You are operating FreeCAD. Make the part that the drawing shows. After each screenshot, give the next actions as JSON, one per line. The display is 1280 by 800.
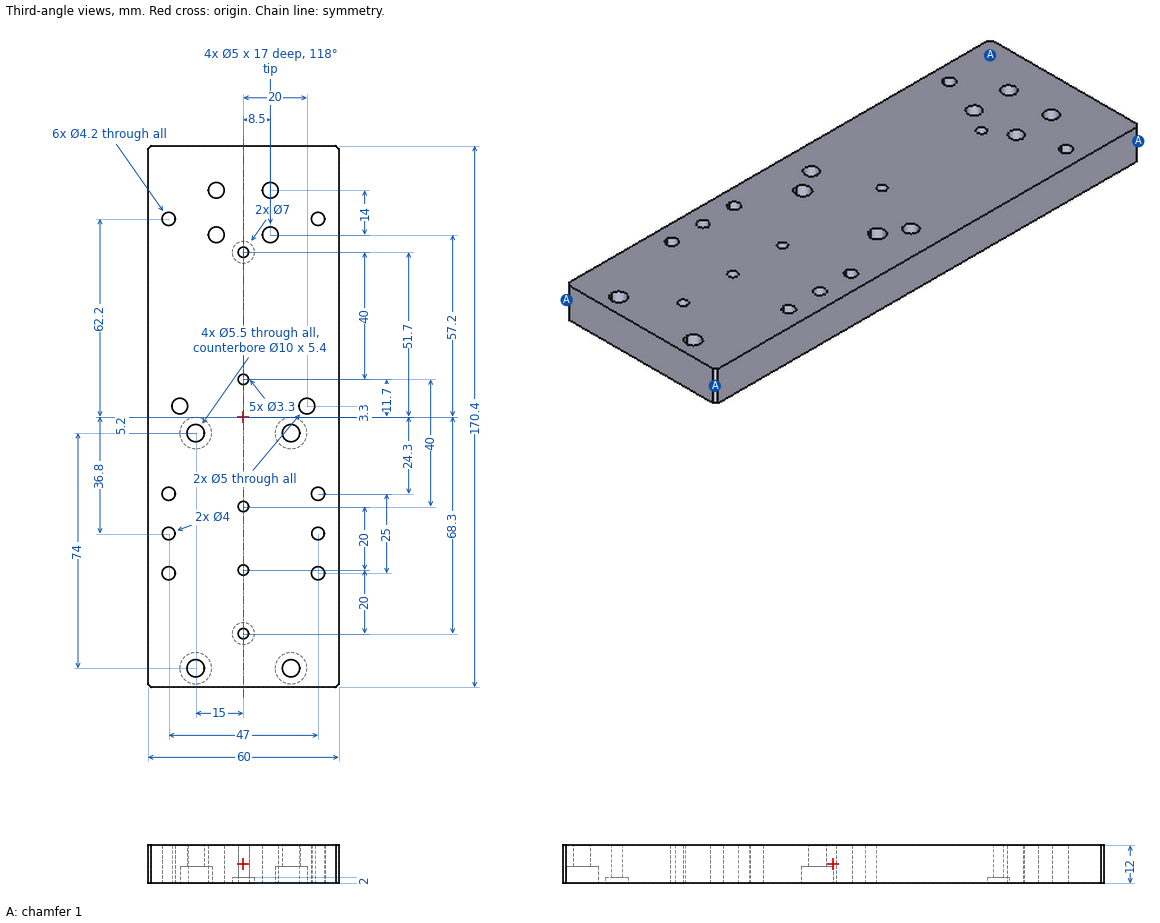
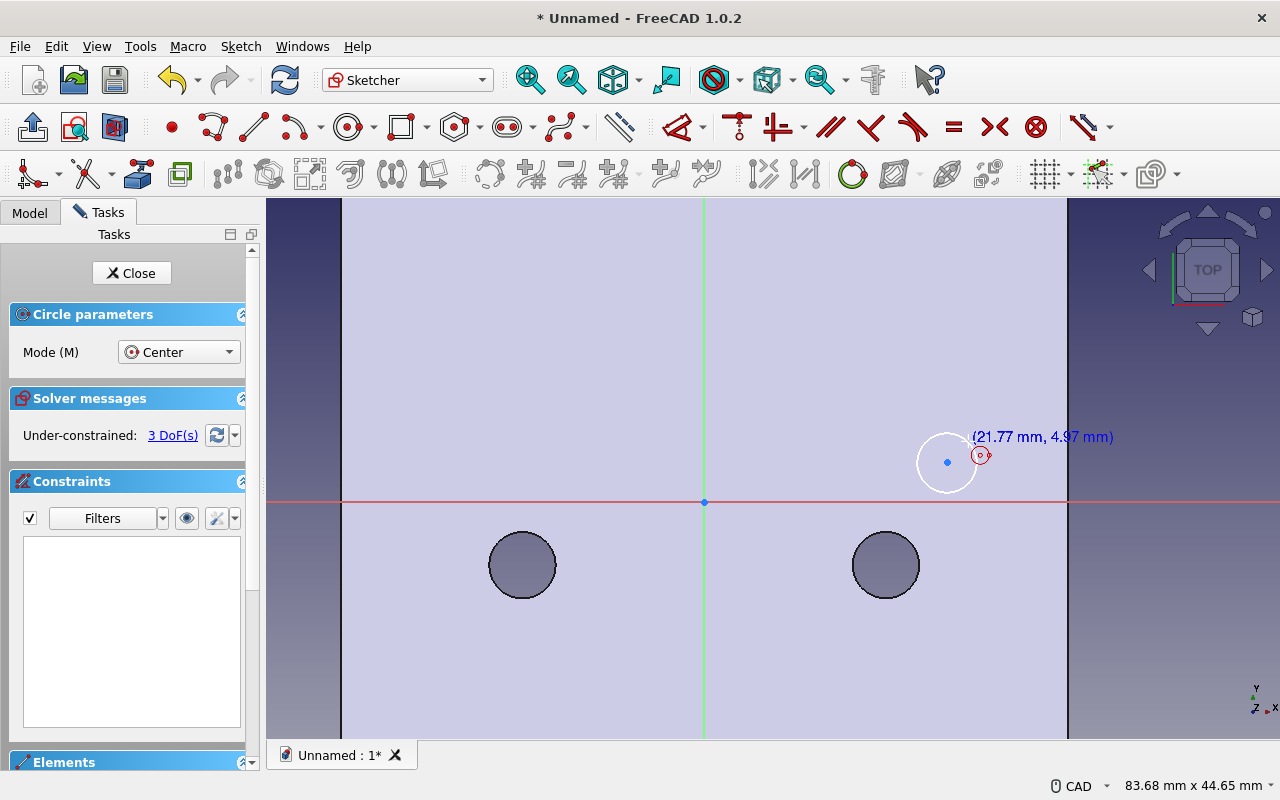
{"action": "left_click", "coordinate": [462, 462]}
{"action": "left_click", "coordinate": [483, 441]}
{"action": "key", "text": "Escape"}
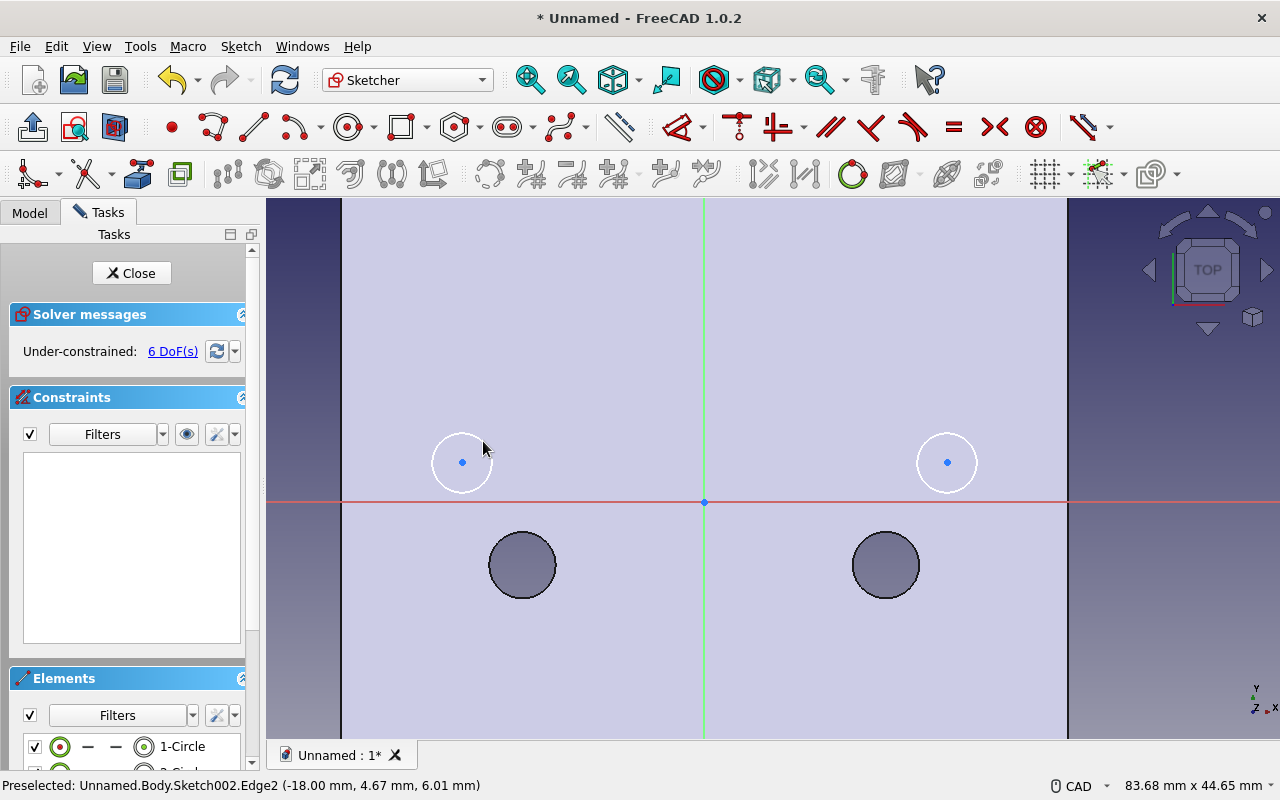
{"action": "left_click", "coordinate": [968, 442]}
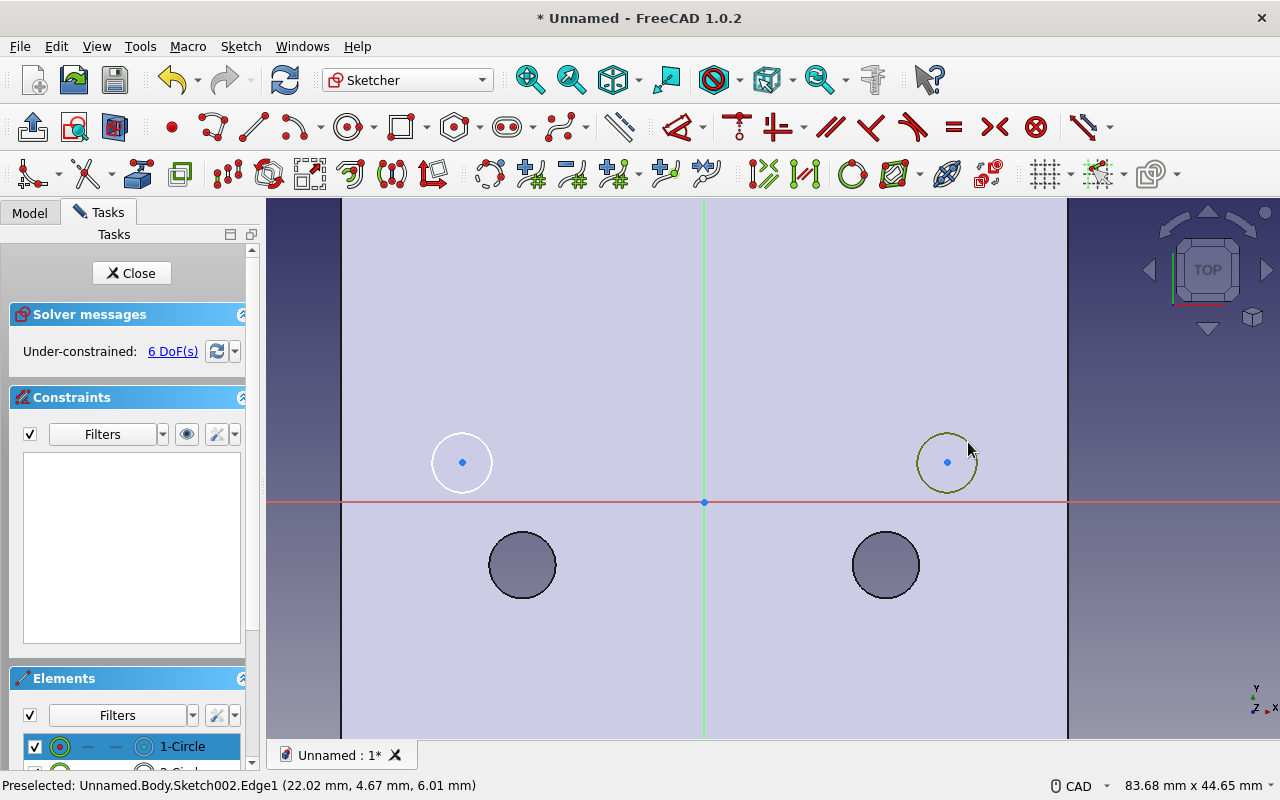
{"action": "left_click", "coordinate": [483, 442]}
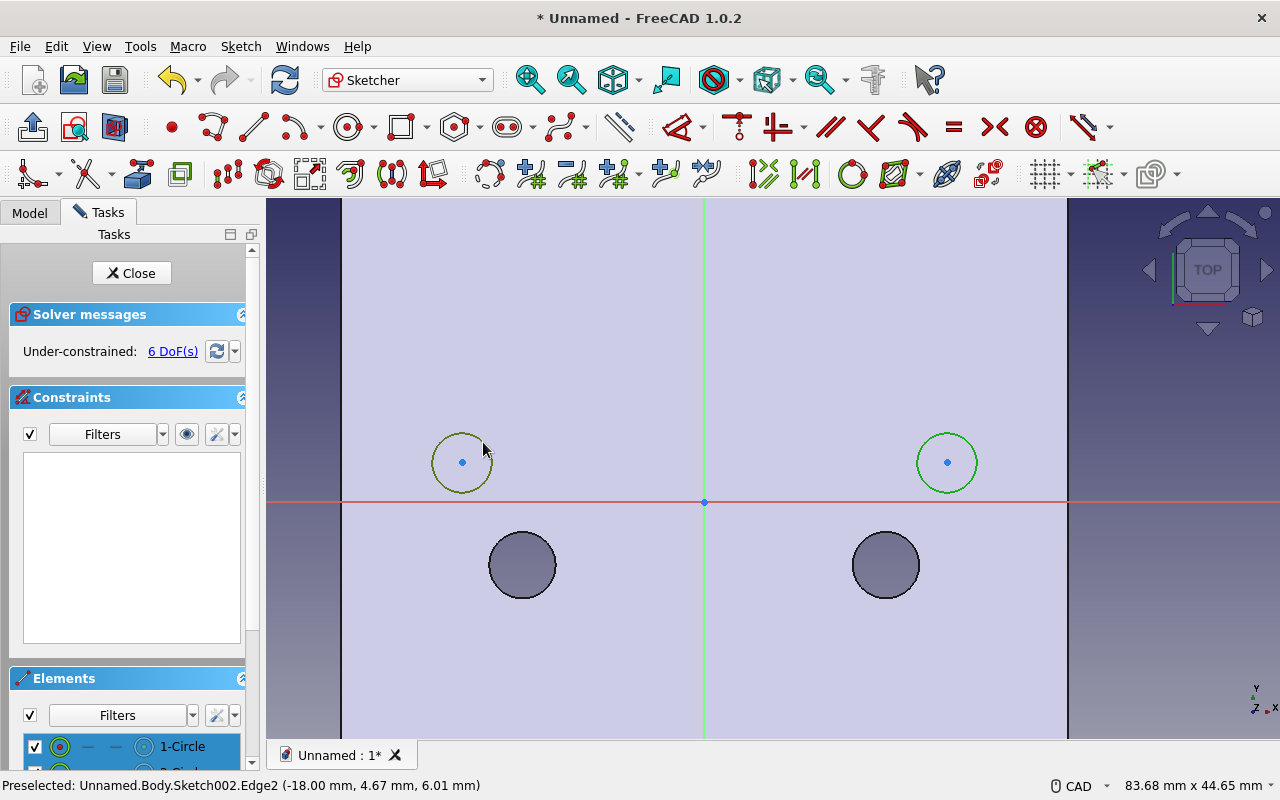
{"action": "left_click", "coordinate": [954, 128]}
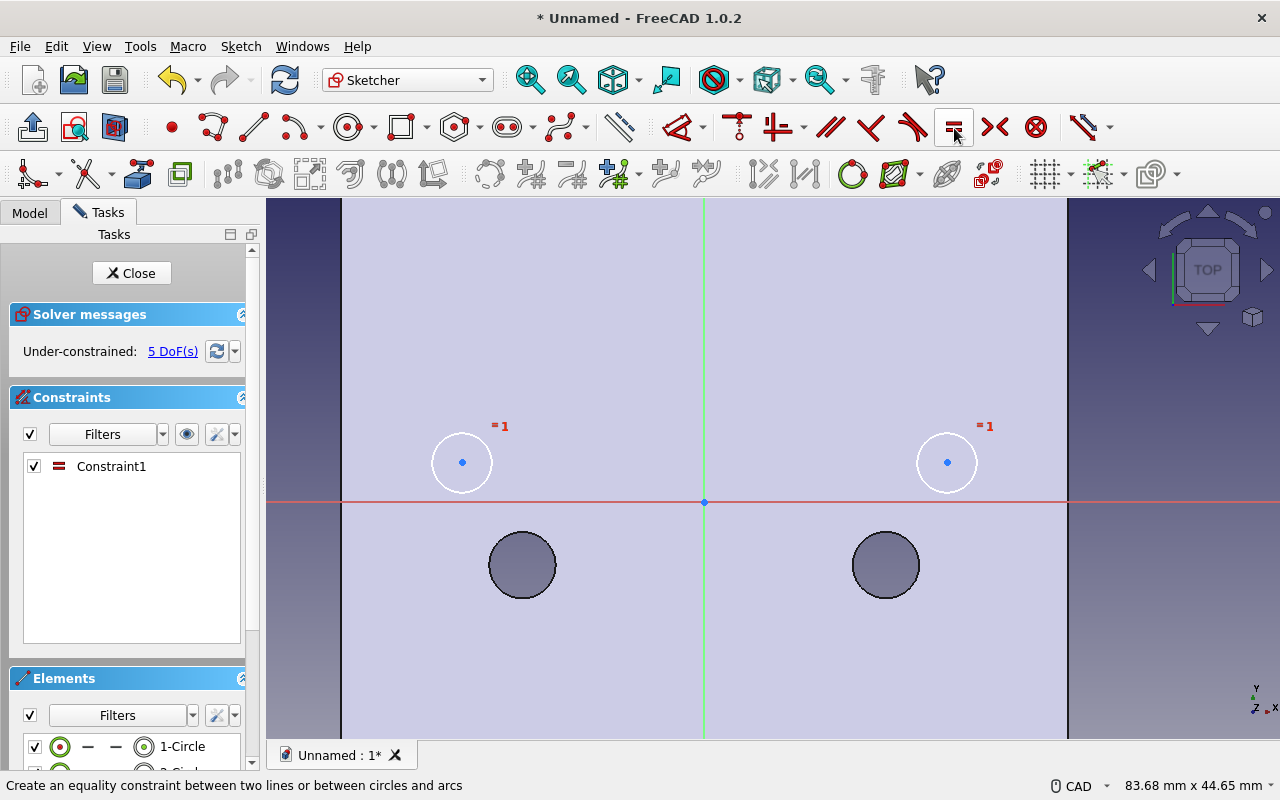
{"action": "left_click", "coordinate": [947, 463]}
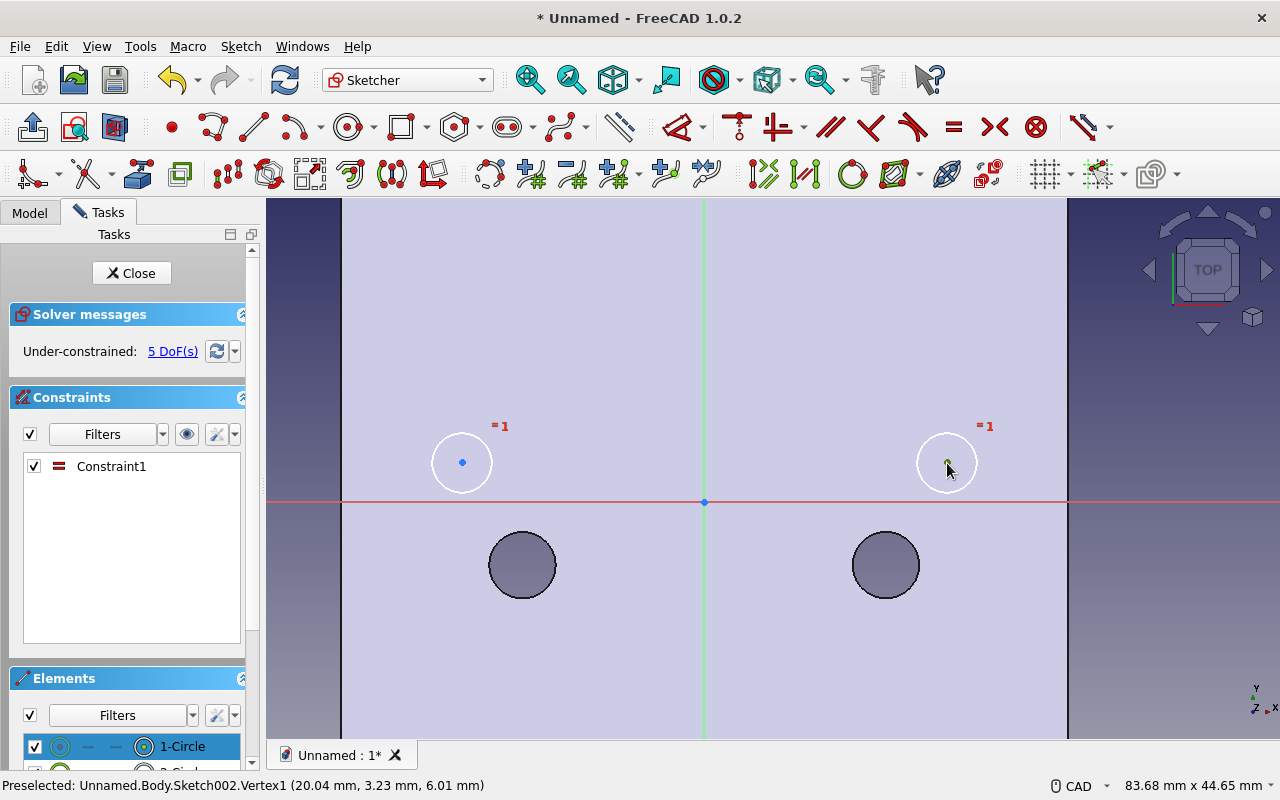
{"action": "left_click", "coordinate": [462, 463]}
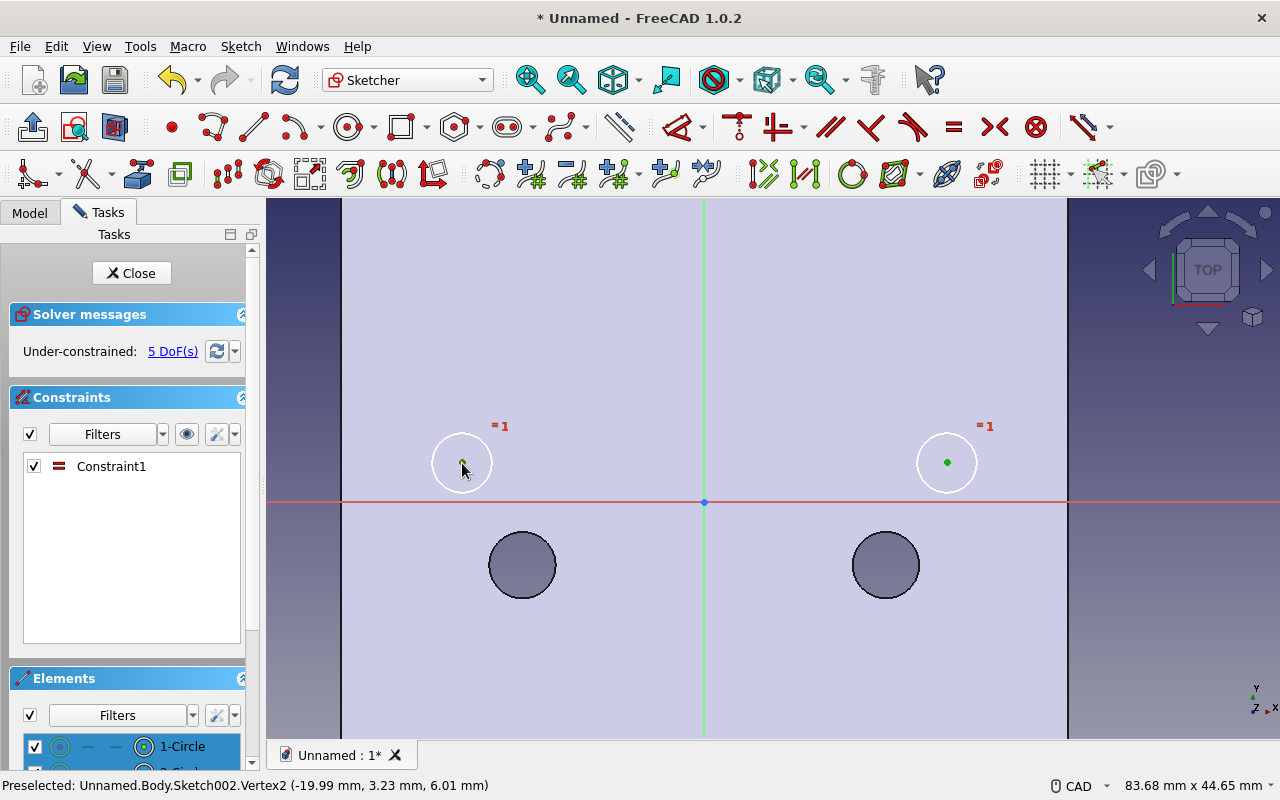
{"action": "left_click", "coordinate": [704, 676]}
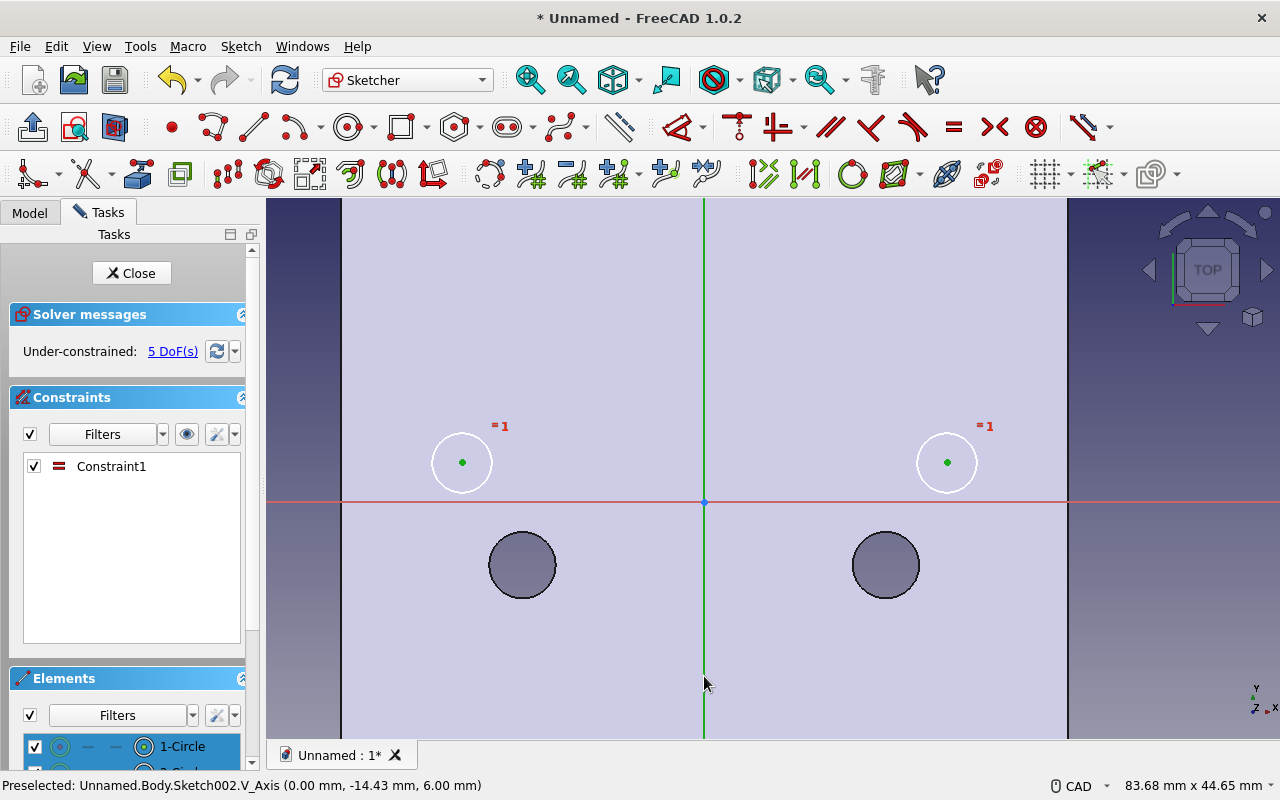
{"action": "left_click", "coordinate": [995, 128]}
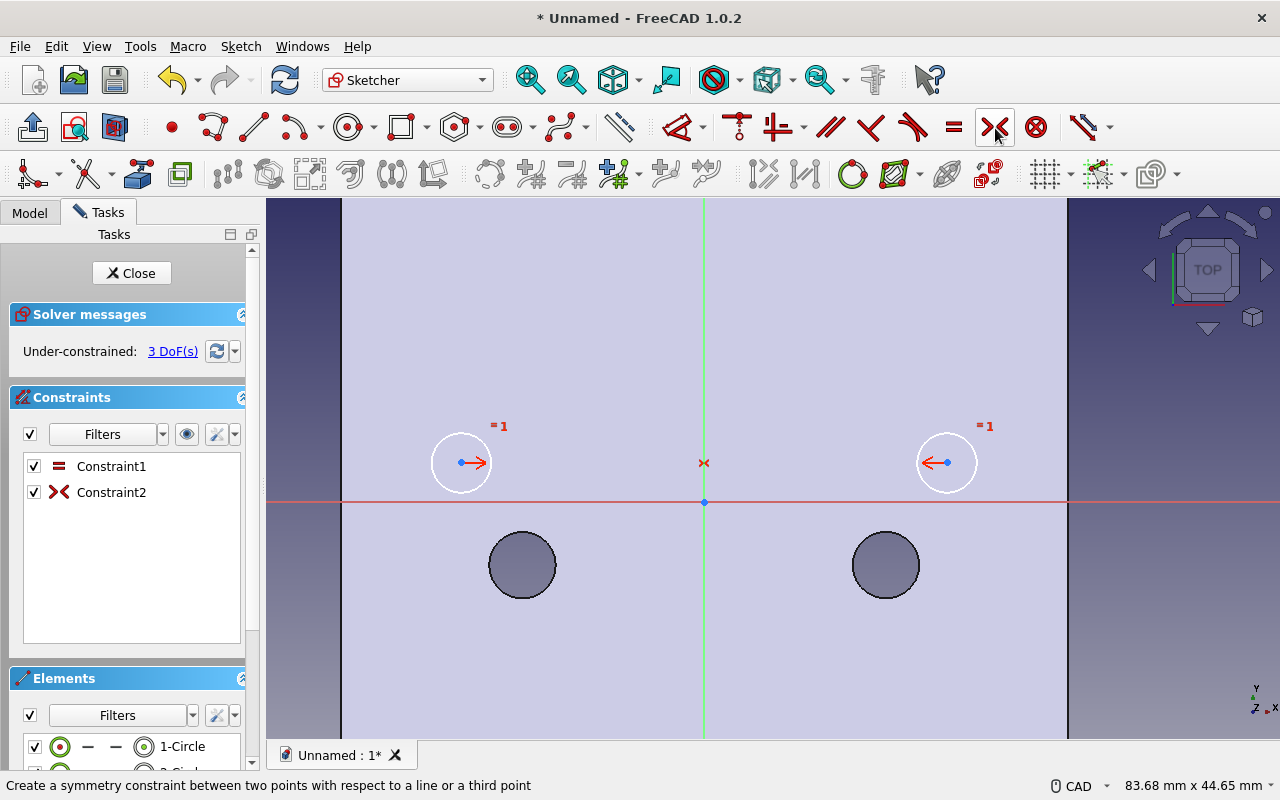
{"action": "left_click", "coordinate": [676, 128]}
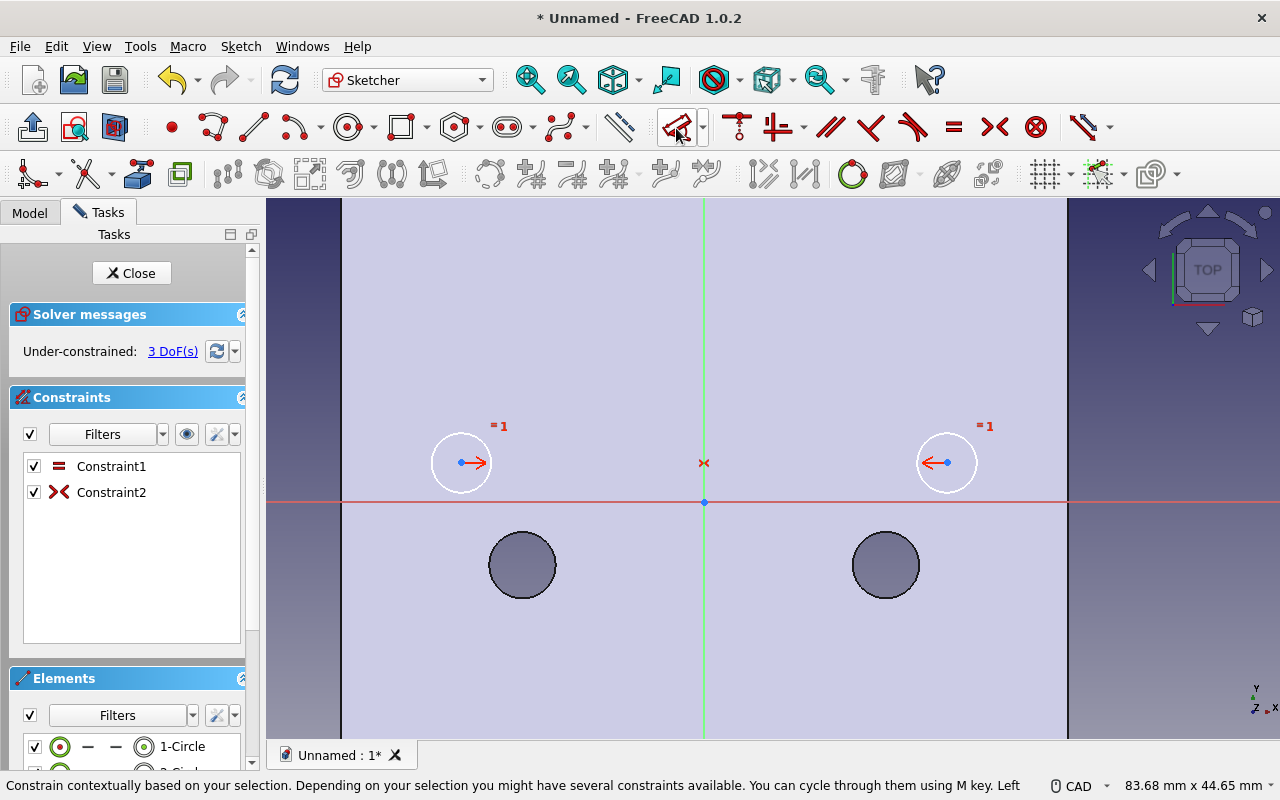
{"action": "left_click", "coordinate": [968, 442]}
{"action": "left_click", "coordinate": [991, 419]}